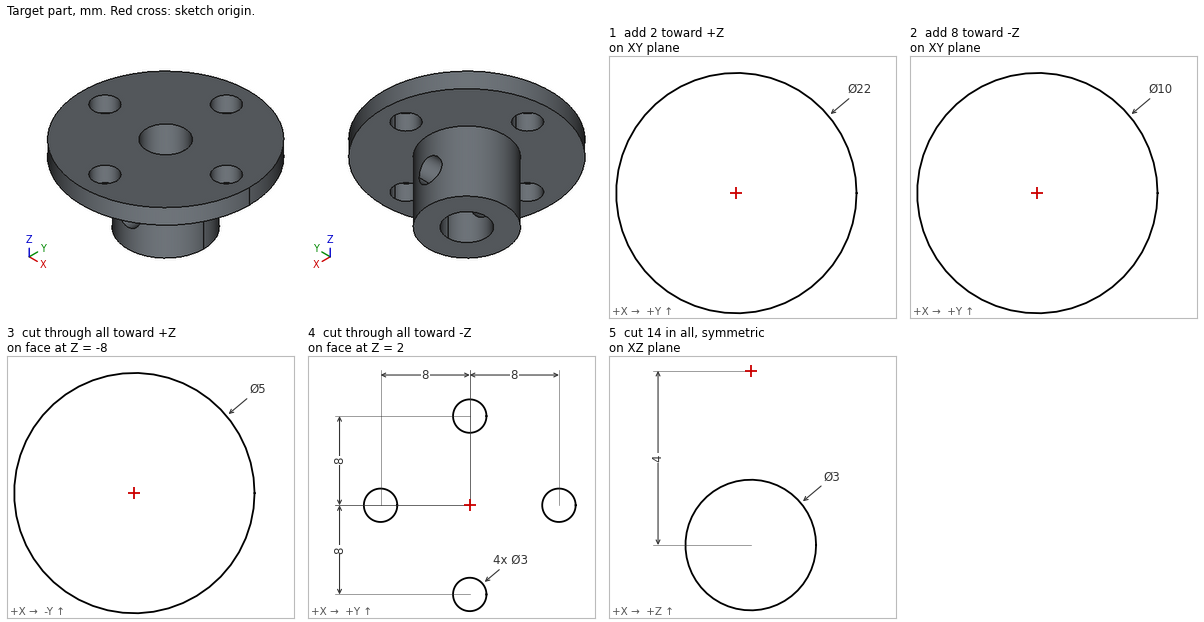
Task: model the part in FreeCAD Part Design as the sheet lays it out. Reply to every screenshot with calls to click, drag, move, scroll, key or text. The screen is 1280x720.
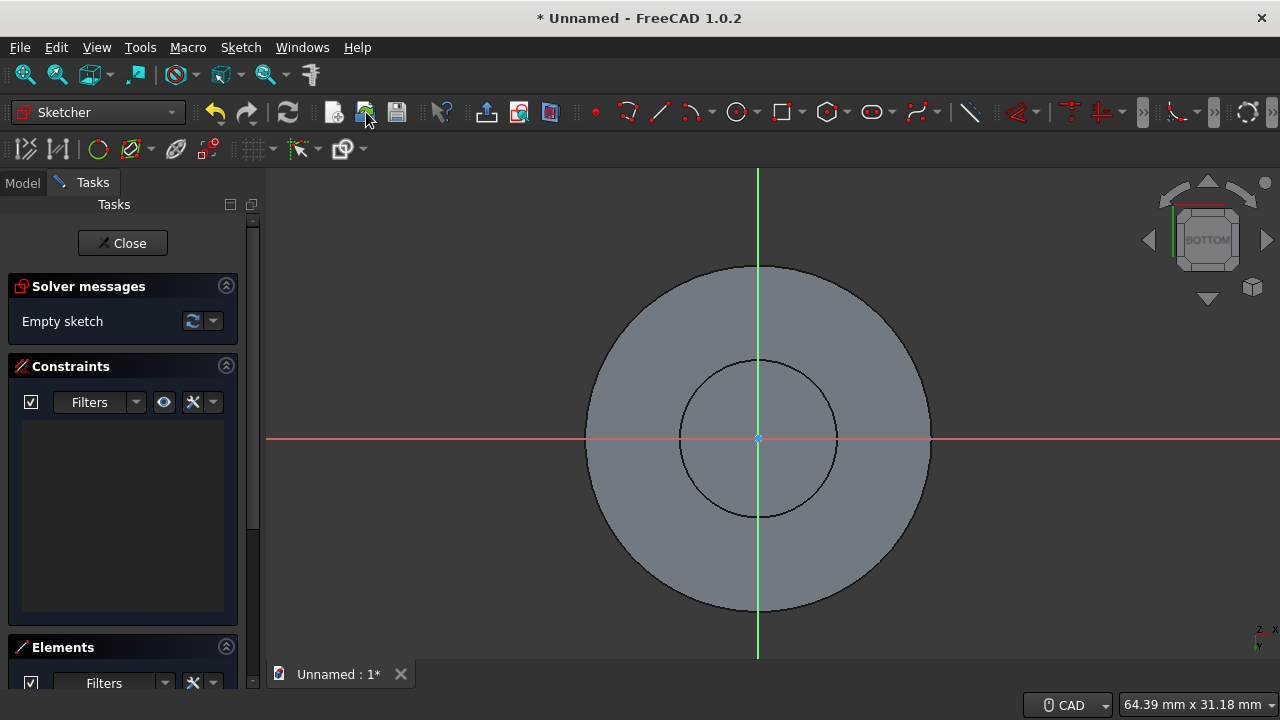
scroll(776, 447, up, 7)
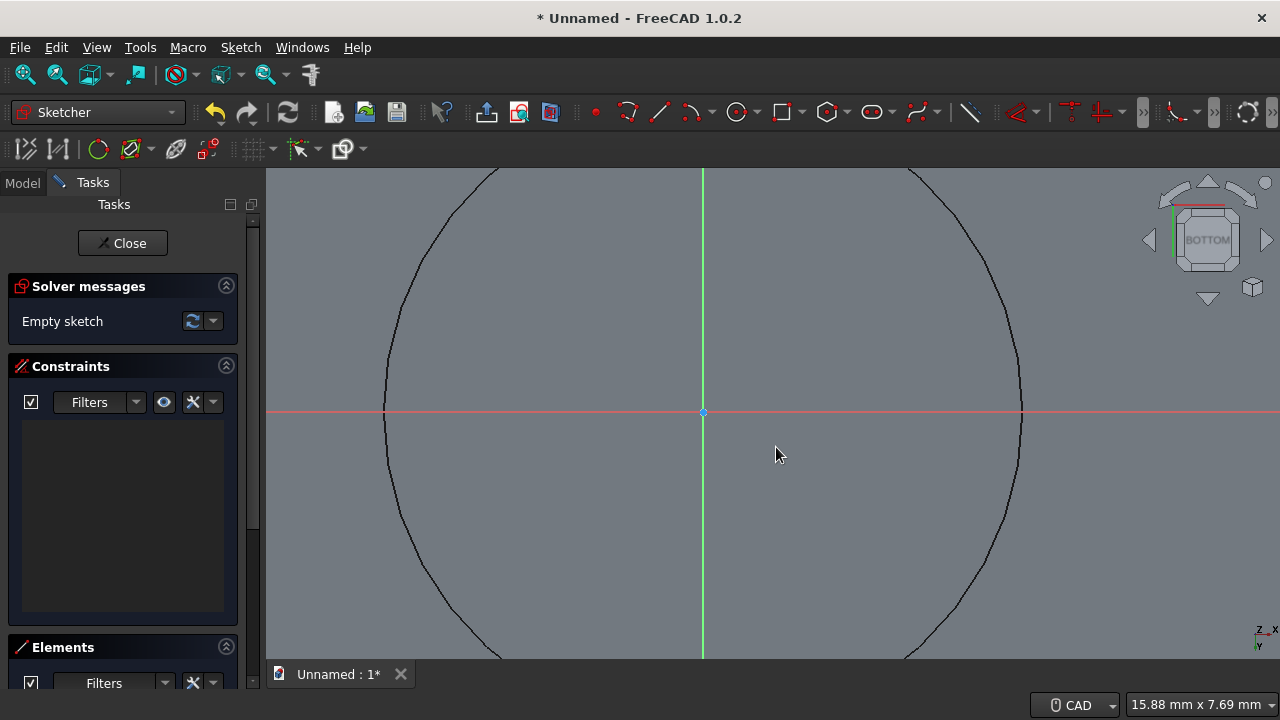
key(g)
key(c)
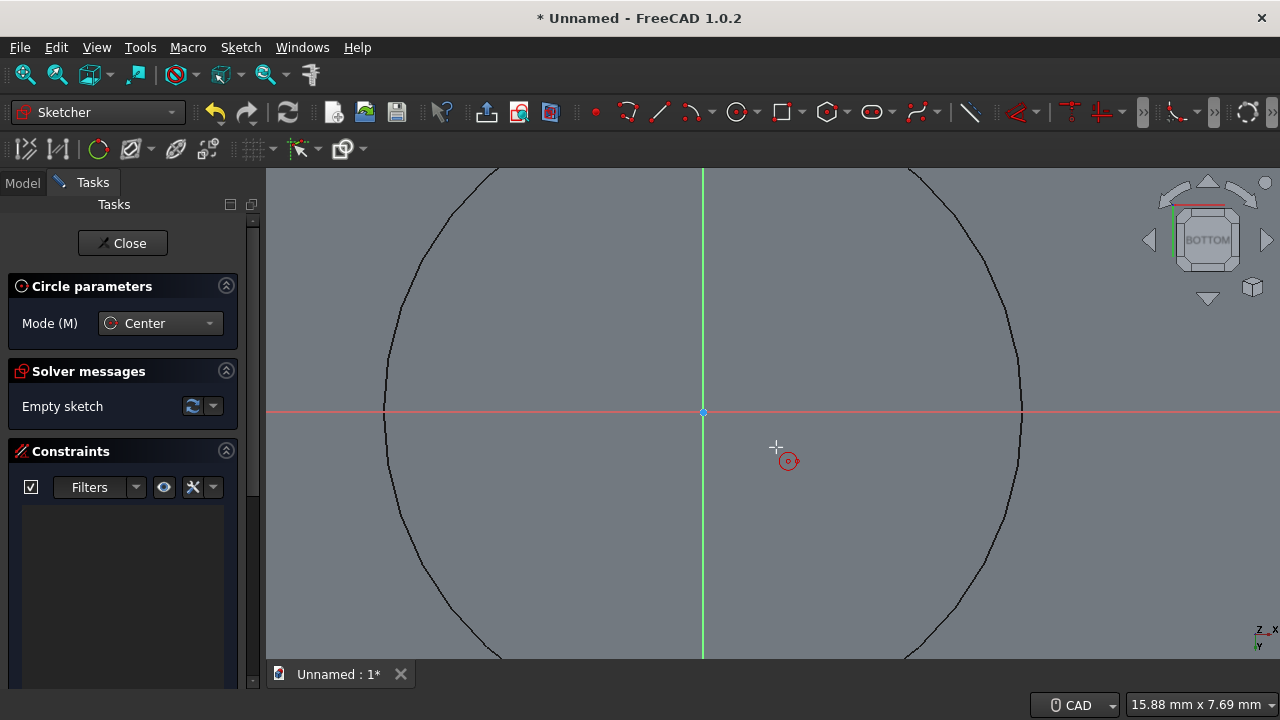
click(703, 412)
click(816, 299)
key(Escape)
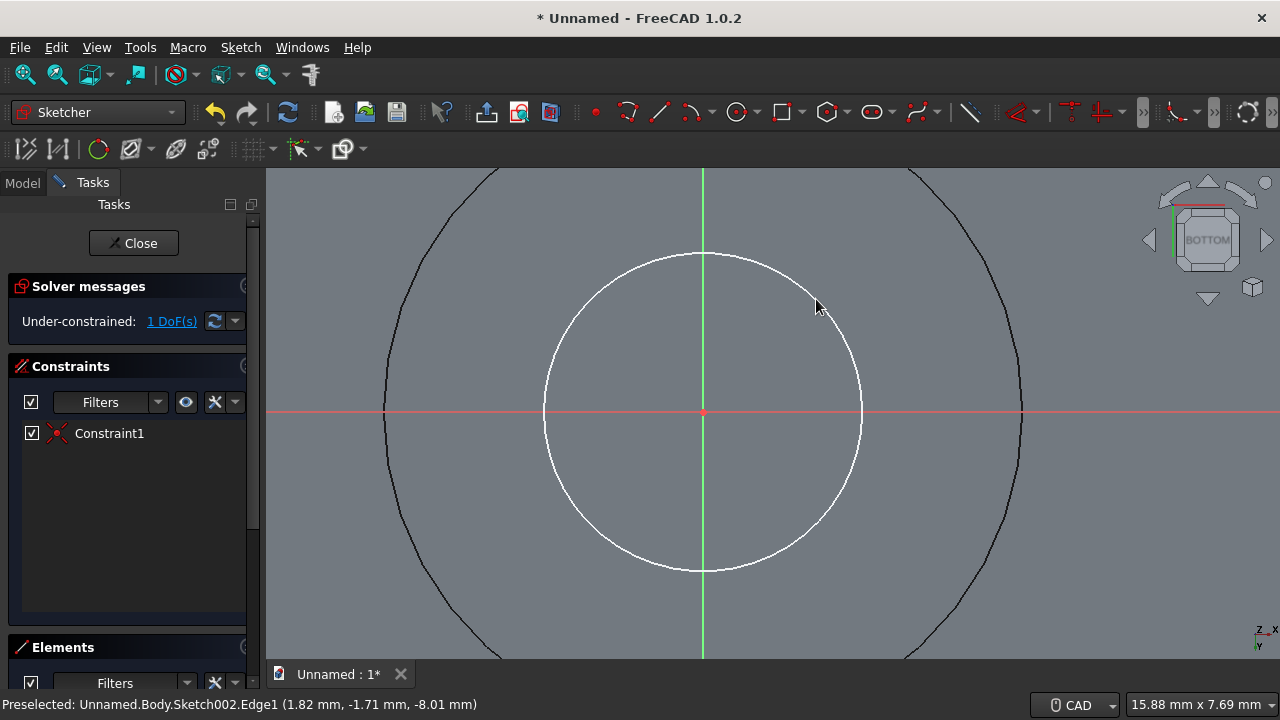
click(815, 299)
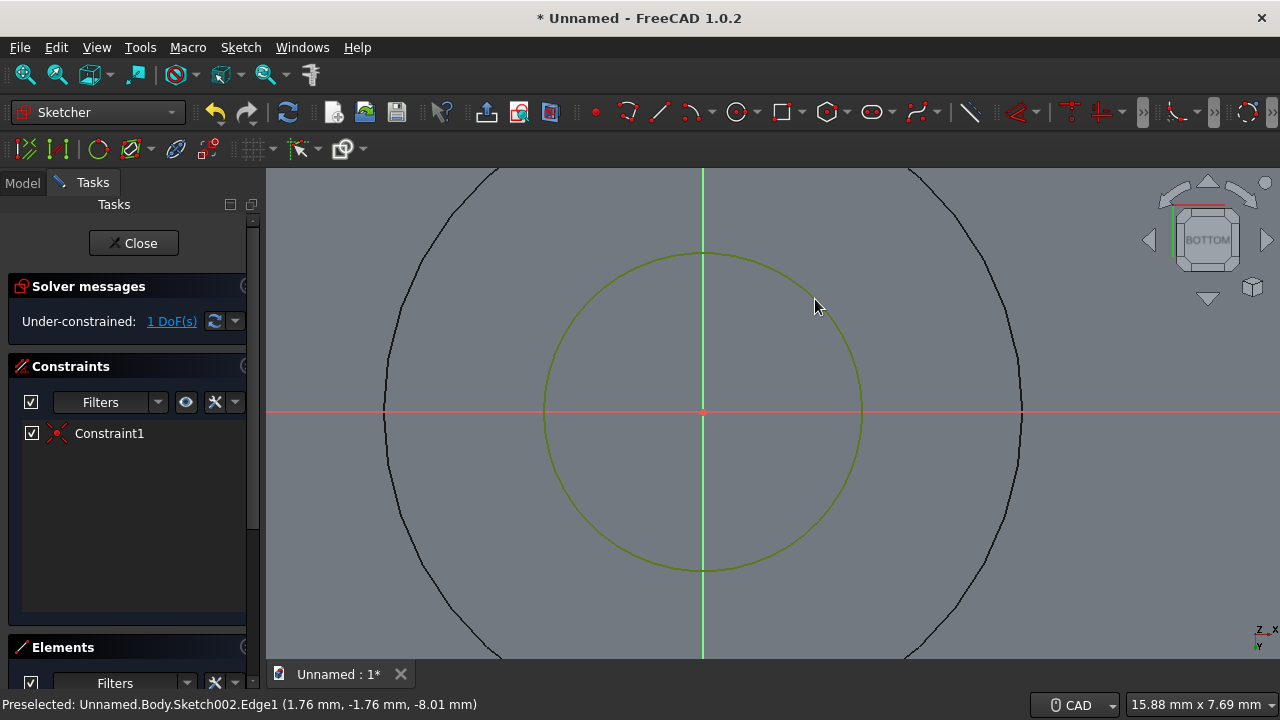
key(k)
key(o)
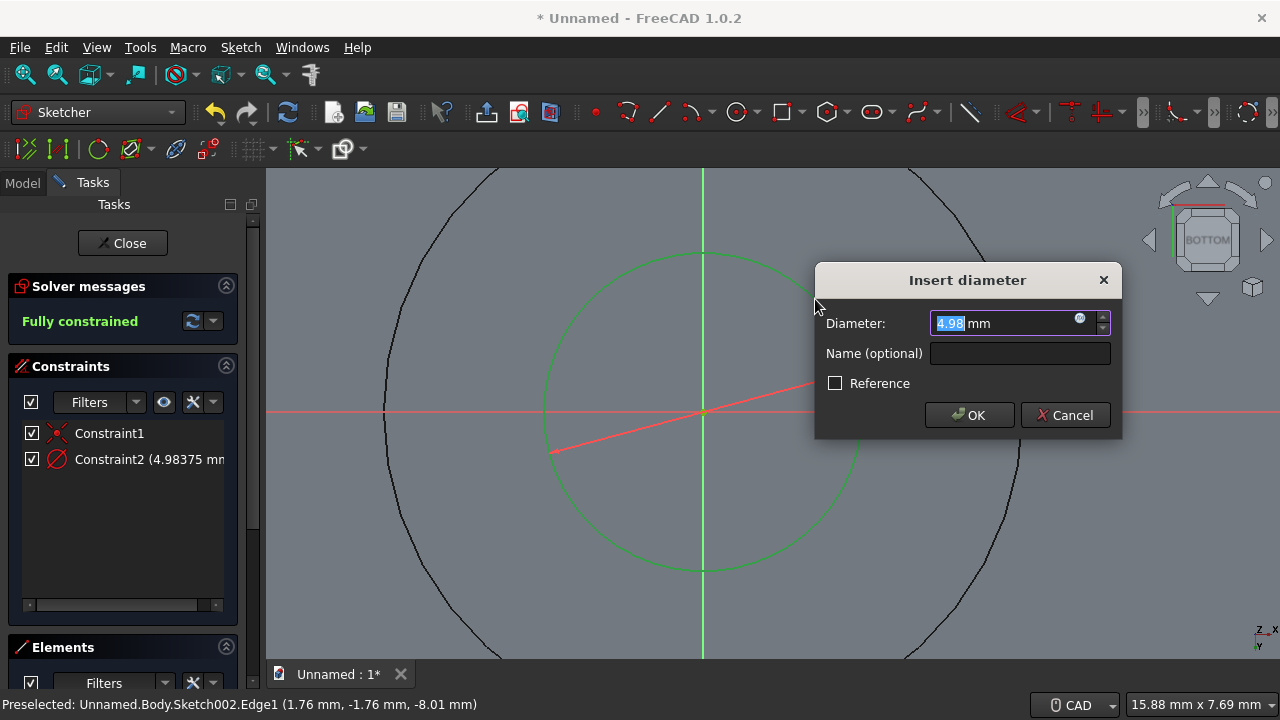
text(5)
key(Return)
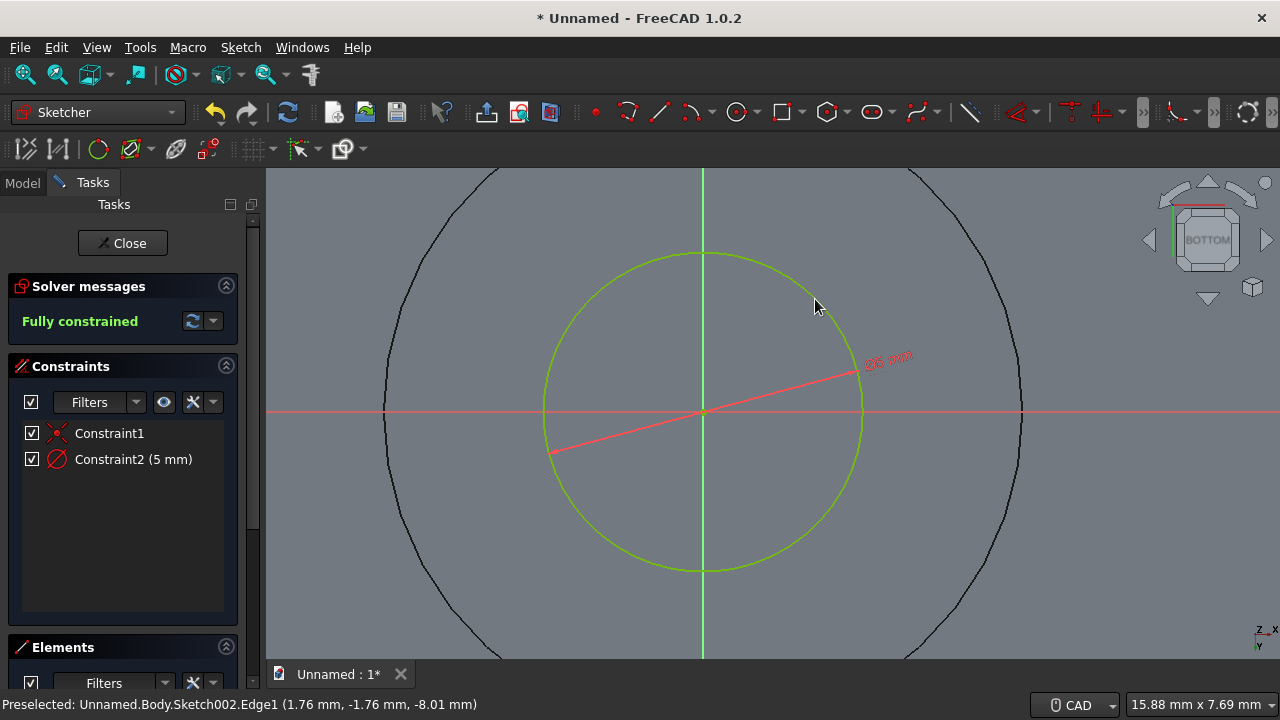
click(123, 243)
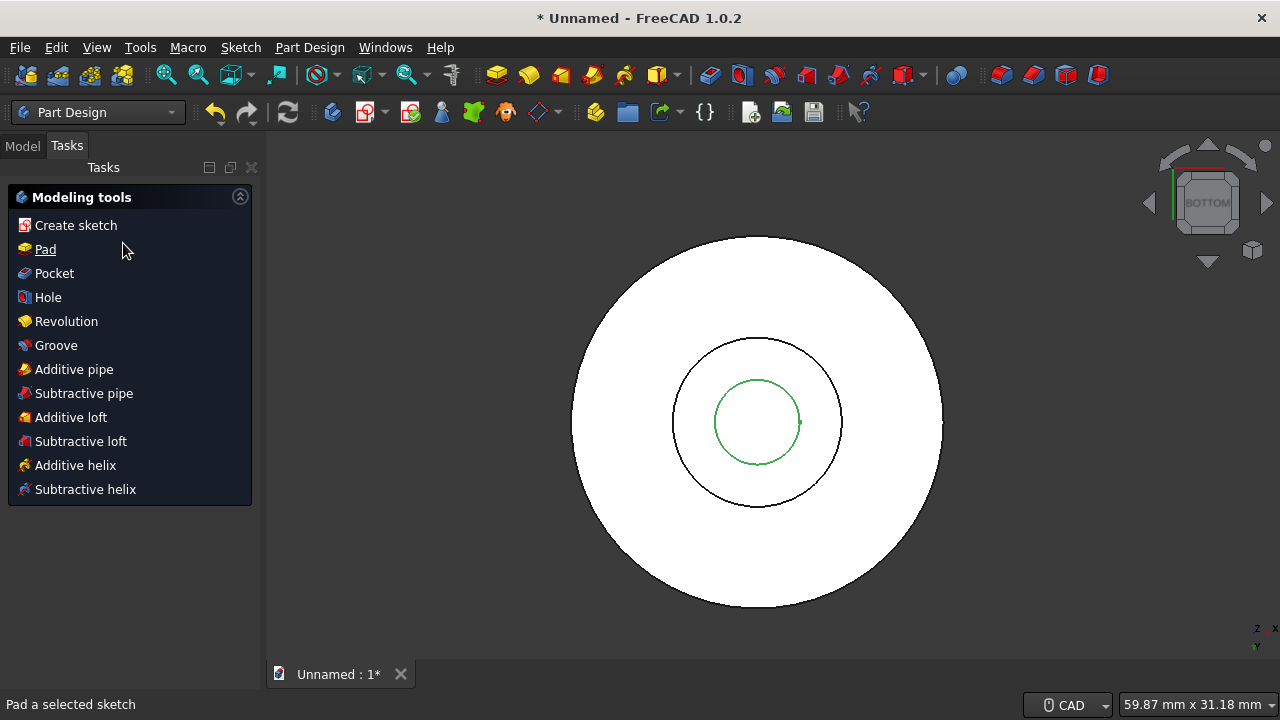
click(712, 76)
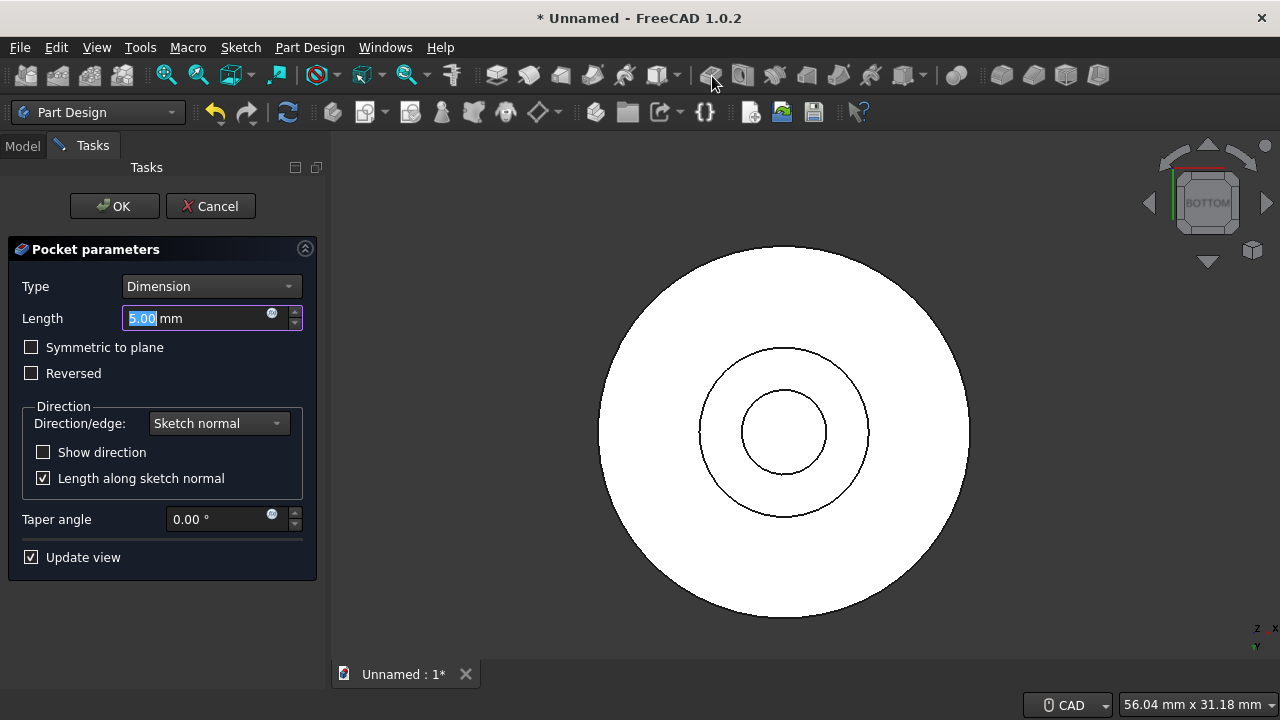
click(212, 286)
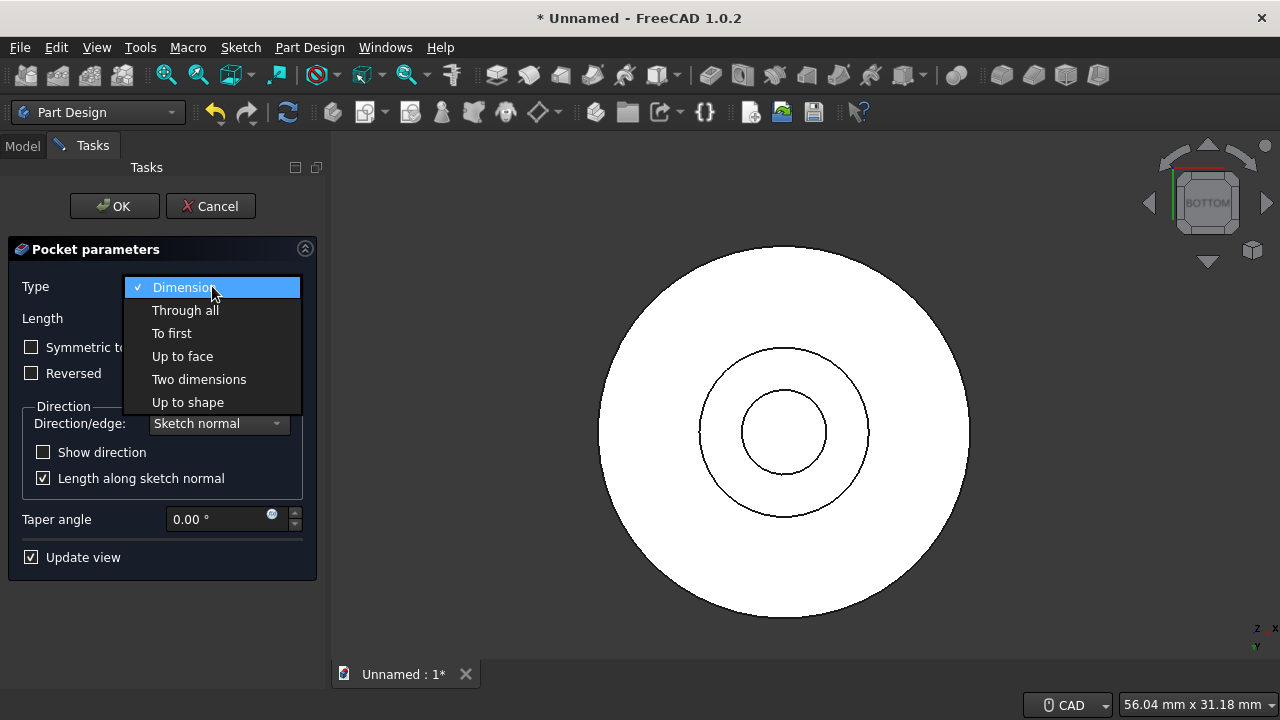
click(212, 310)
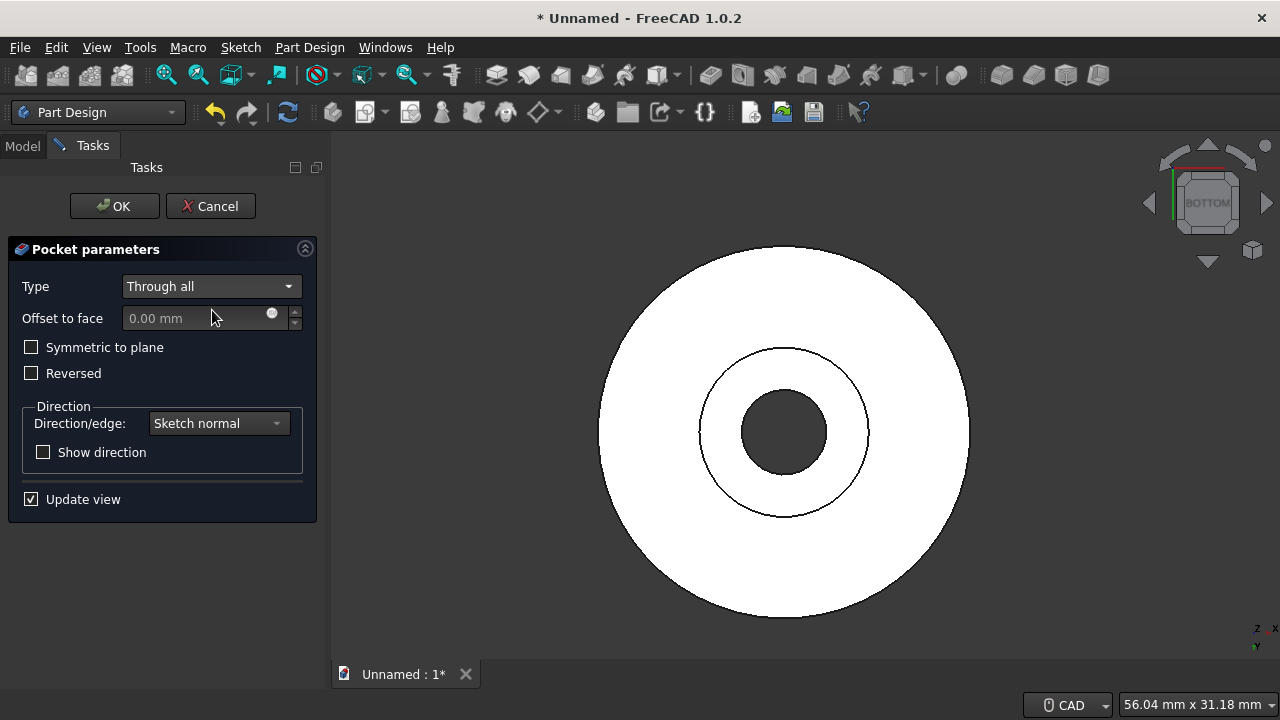
click(115, 206)